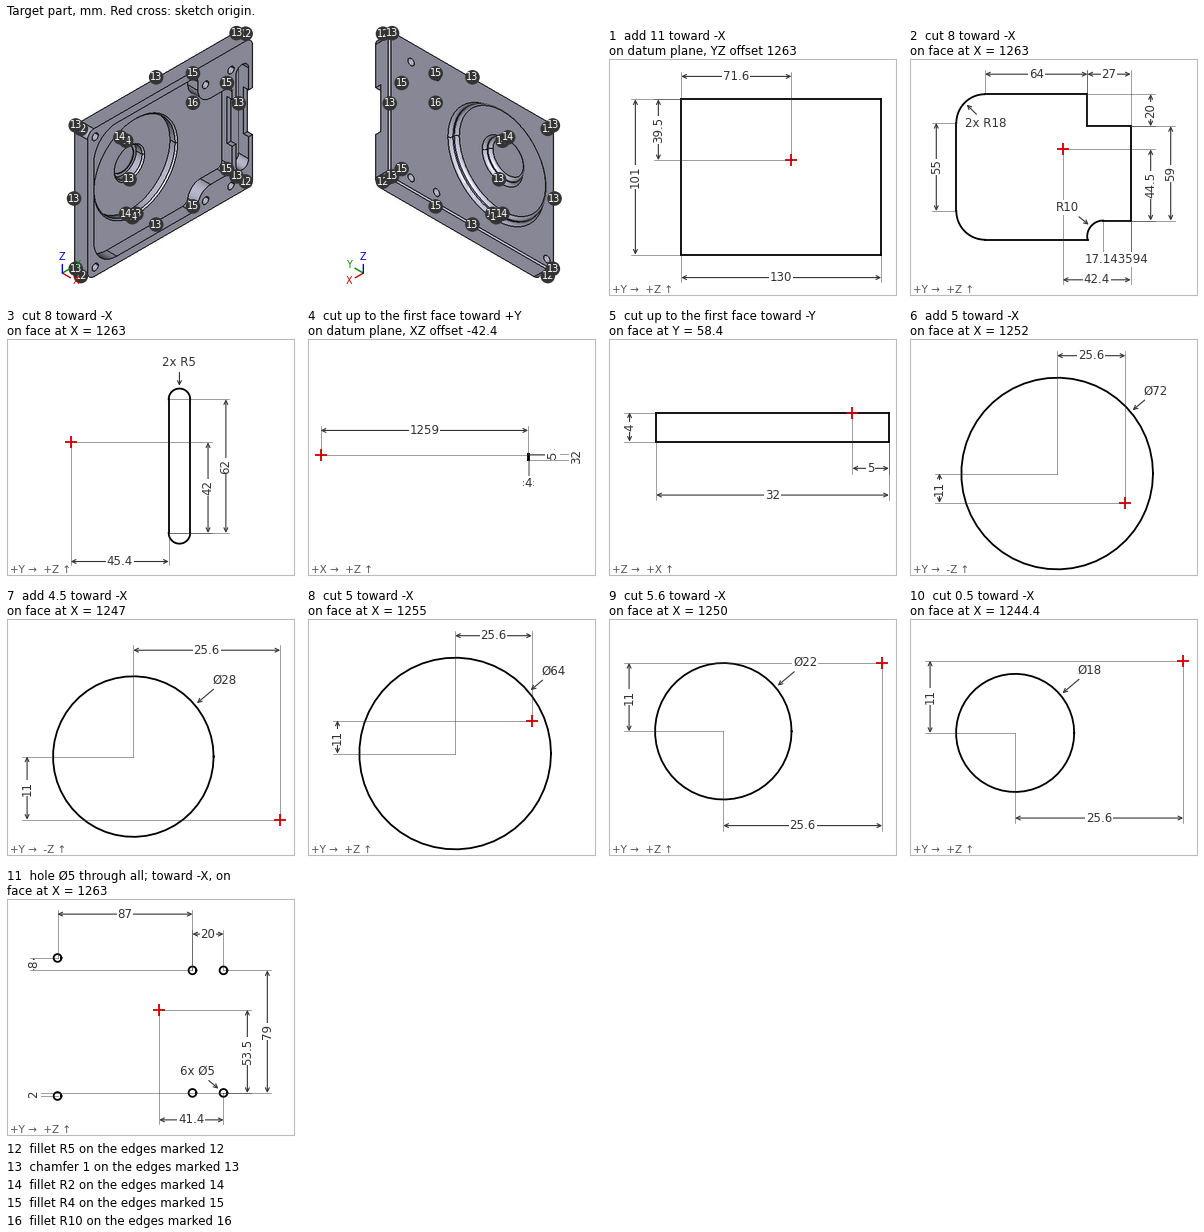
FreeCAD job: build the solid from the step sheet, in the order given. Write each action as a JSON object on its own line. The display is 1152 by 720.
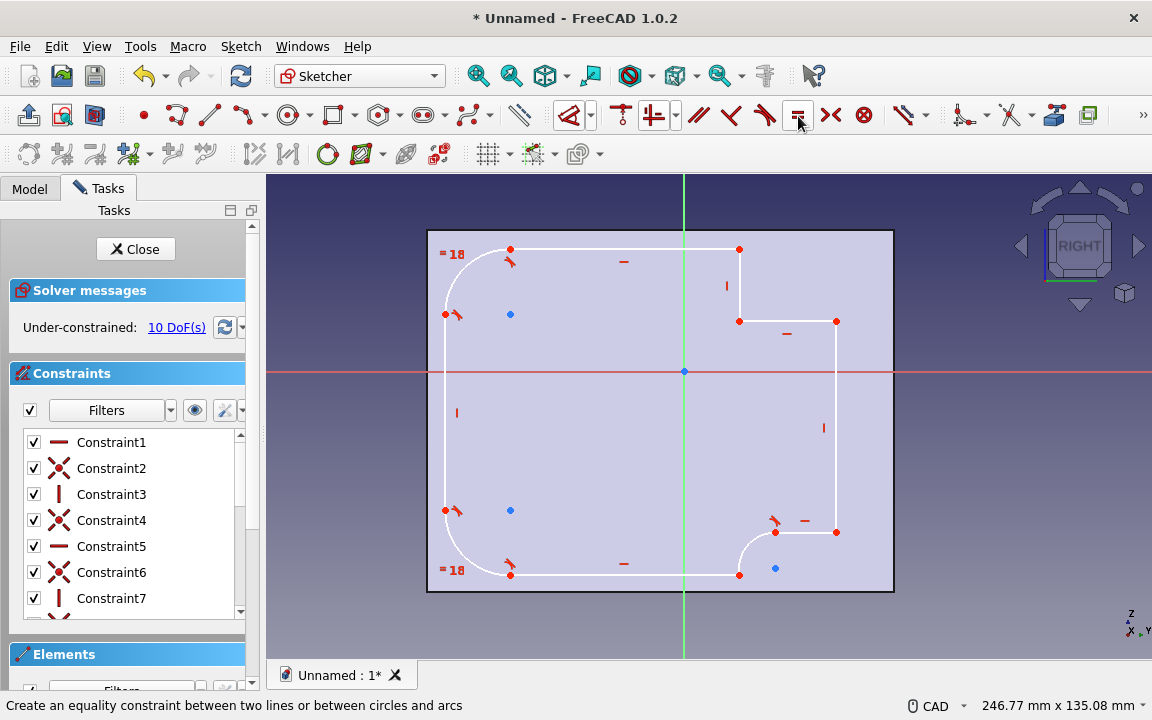
{"action": "left_click", "coordinate": [481, 256]}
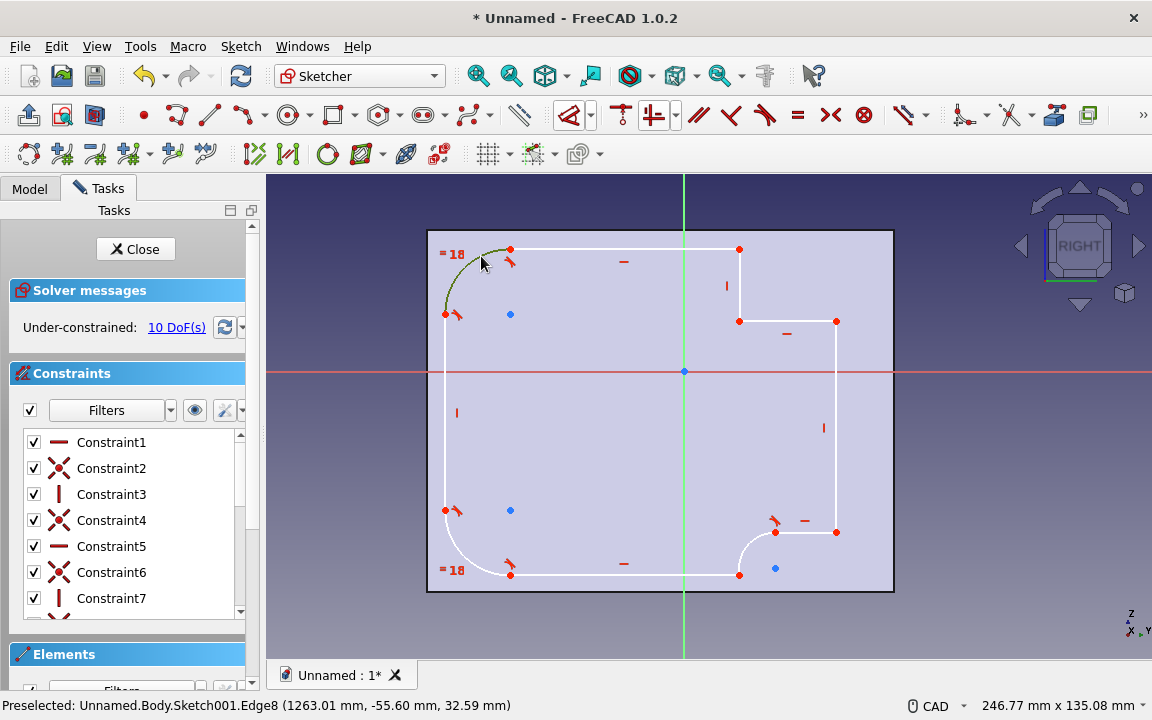
{"action": "left_click", "coordinate": [590, 116]}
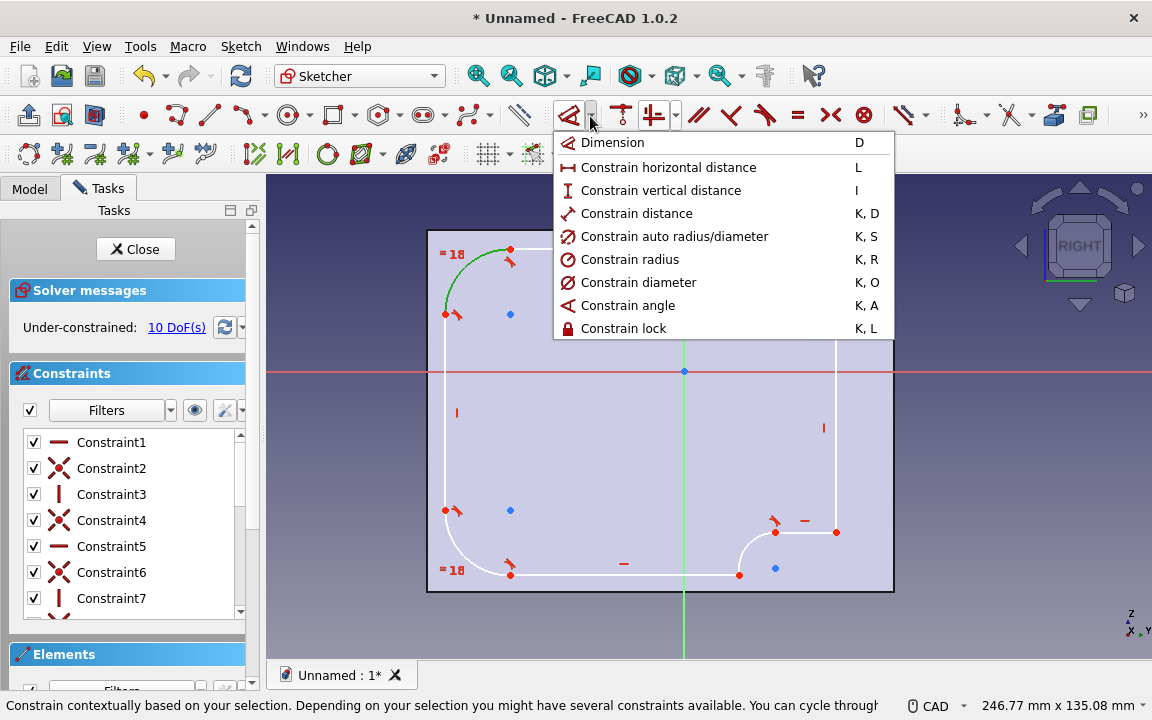
{"action": "left_click", "coordinate": [724, 260]}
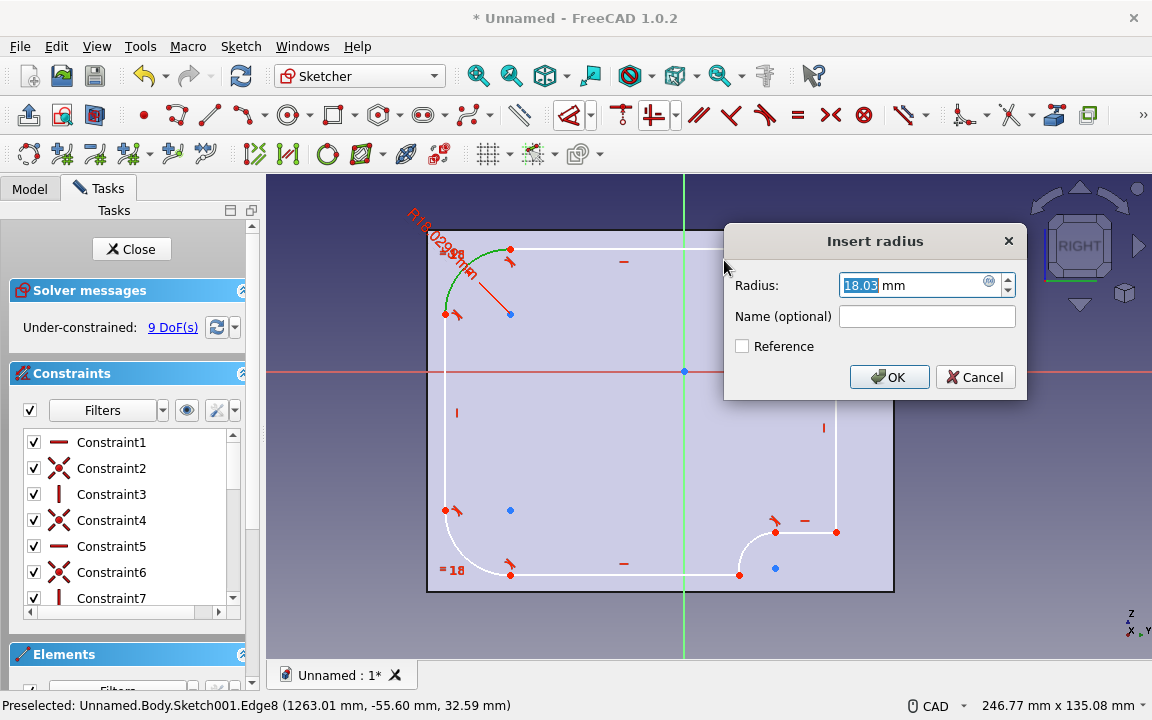
{"action": "type", "text": "18"}
{"action": "key", "text": "Return"}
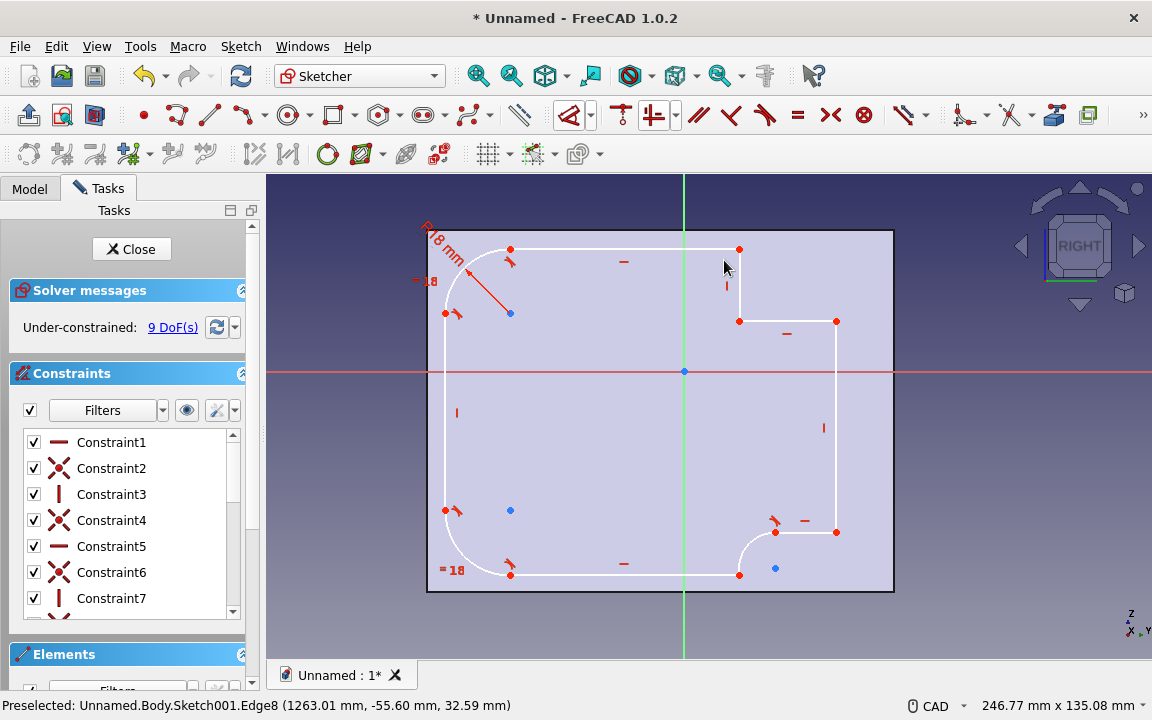
{"action": "left_click", "coordinate": [757, 538]}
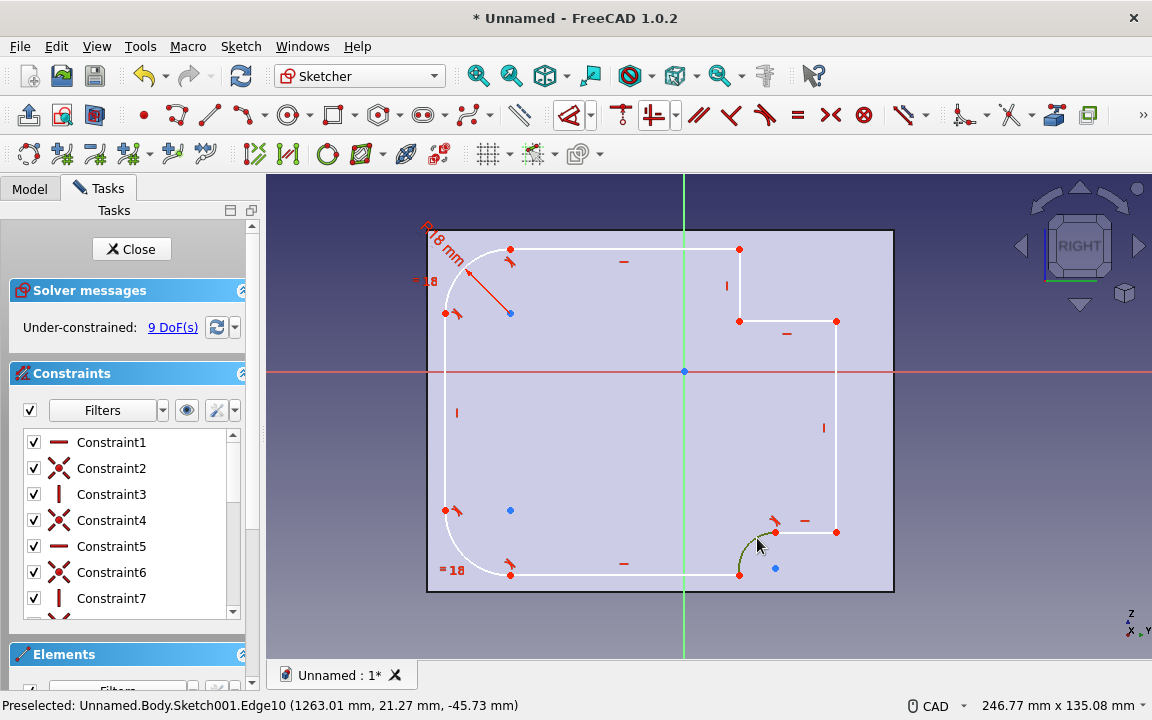
{"action": "left_click", "coordinate": [590, 116]}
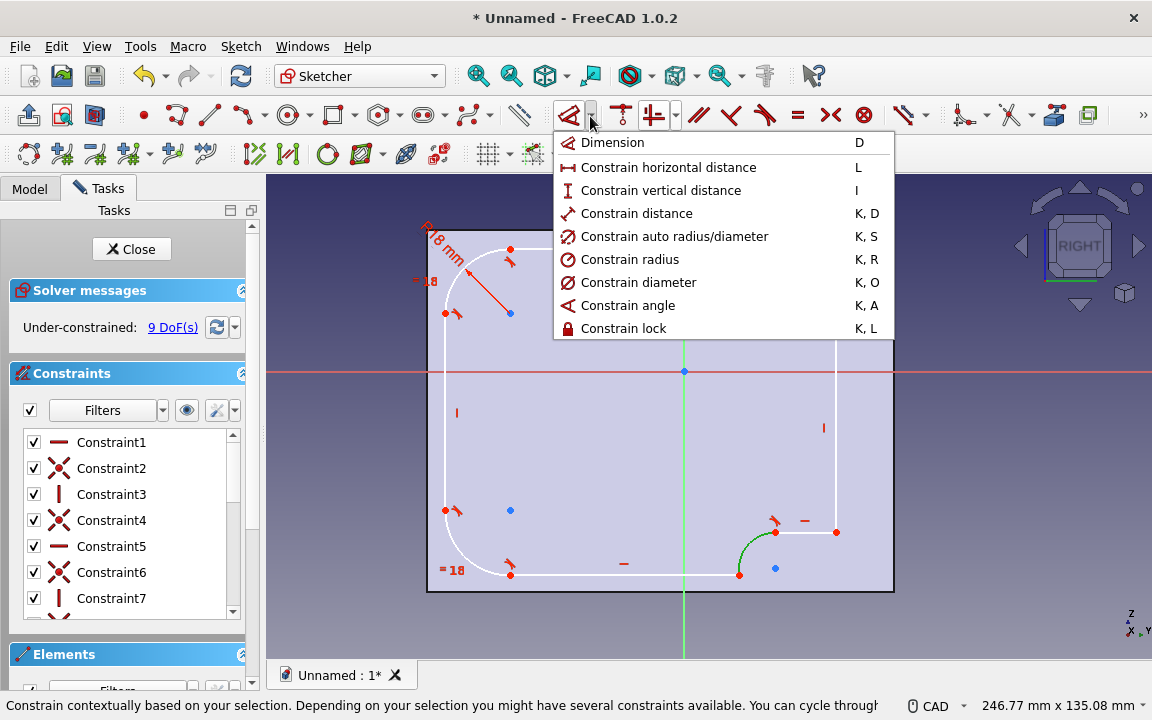
{"action": "left_click", "coordinate": [724, 260]}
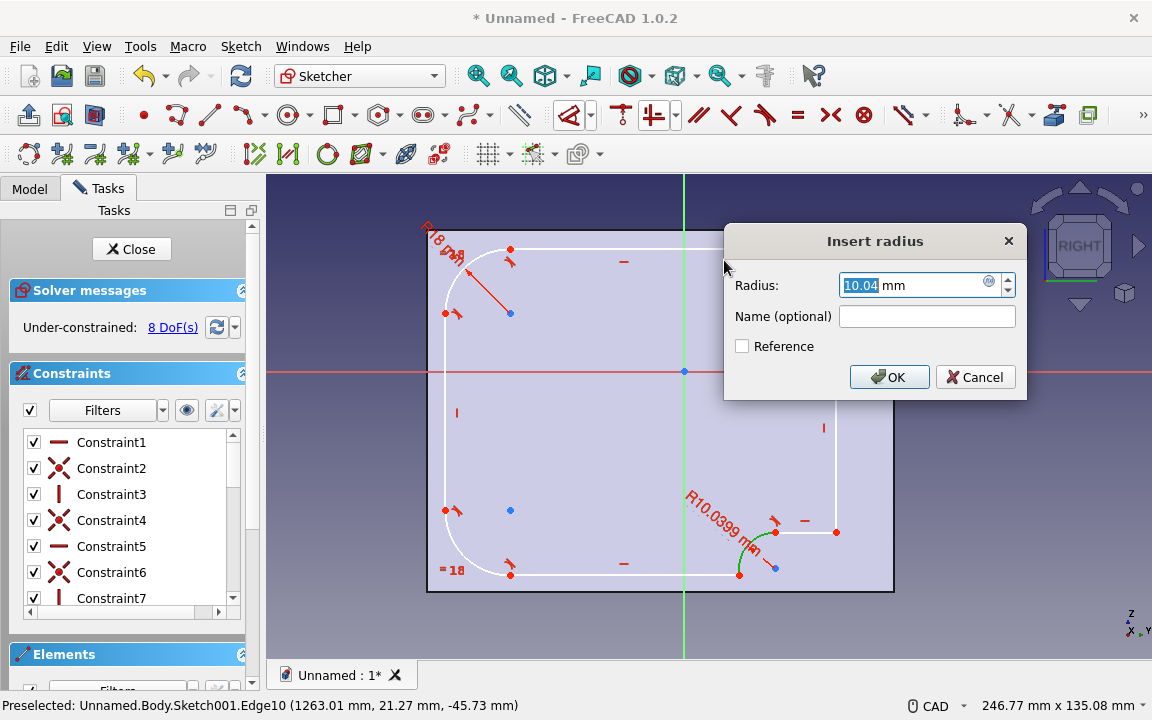
{"action": "type", "text": "10"}
{"action": "key", "text": "Return"}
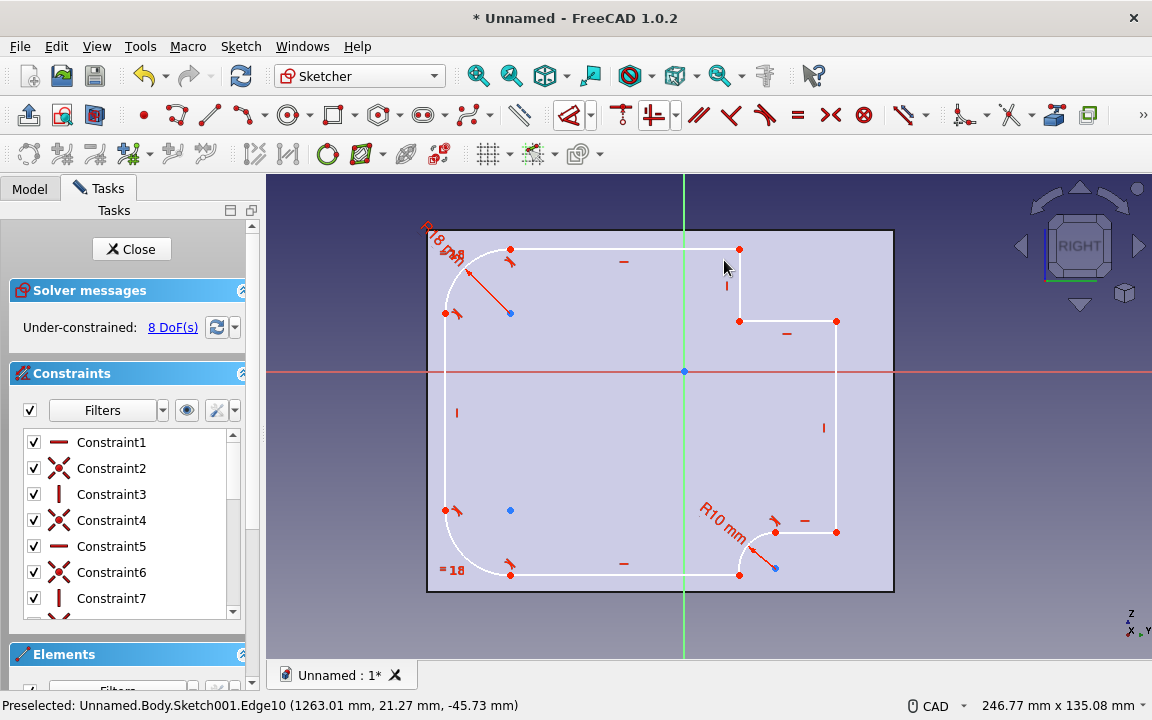
{"action": "left_click", "coordinate": [836, 469]}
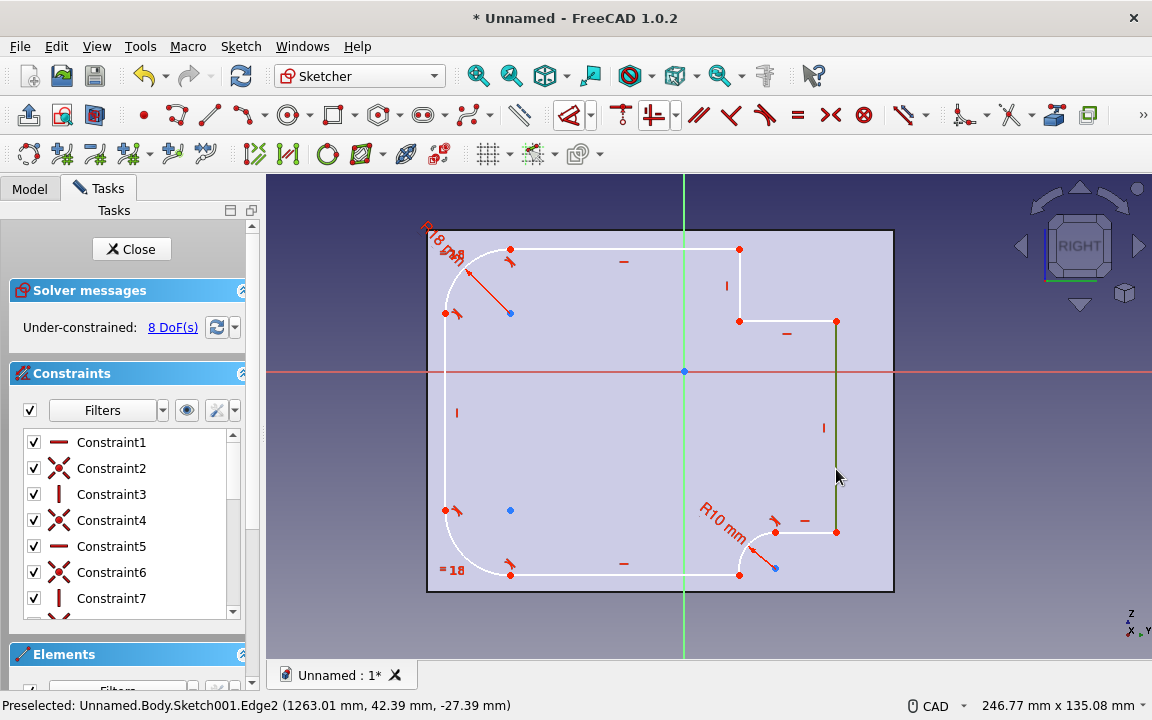
{"action": "left_click", "coordinate": [590, 116]}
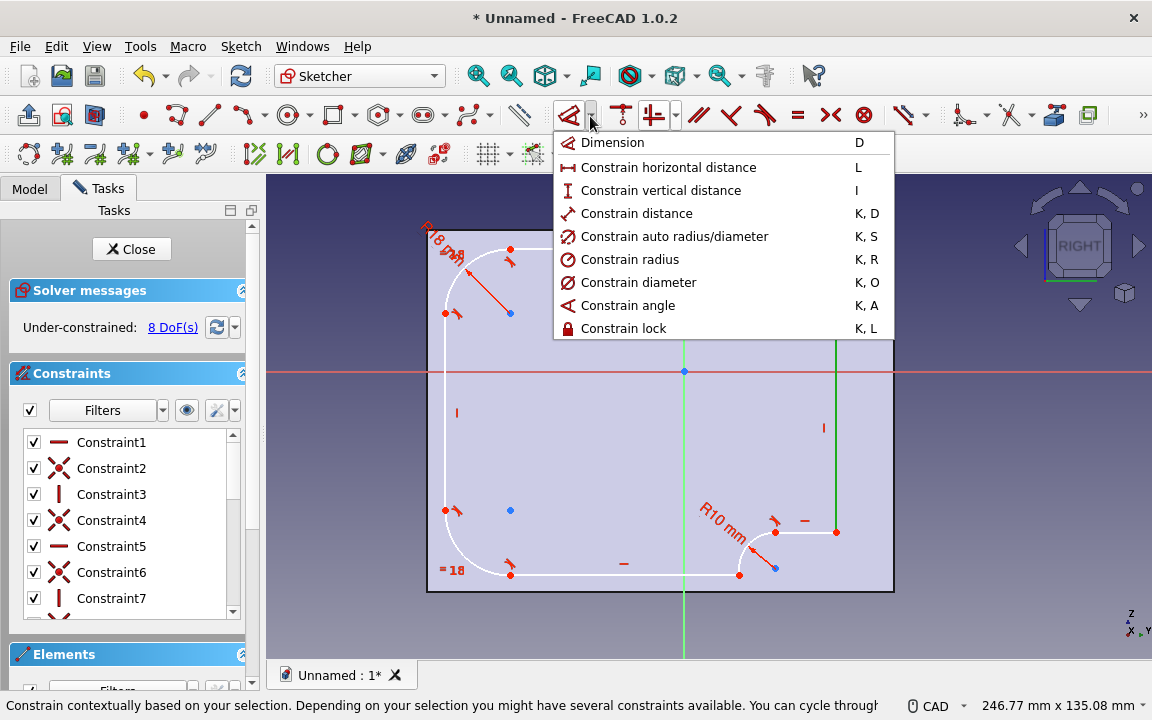
{"action": "left_click", "coordinate": [724, 190]}